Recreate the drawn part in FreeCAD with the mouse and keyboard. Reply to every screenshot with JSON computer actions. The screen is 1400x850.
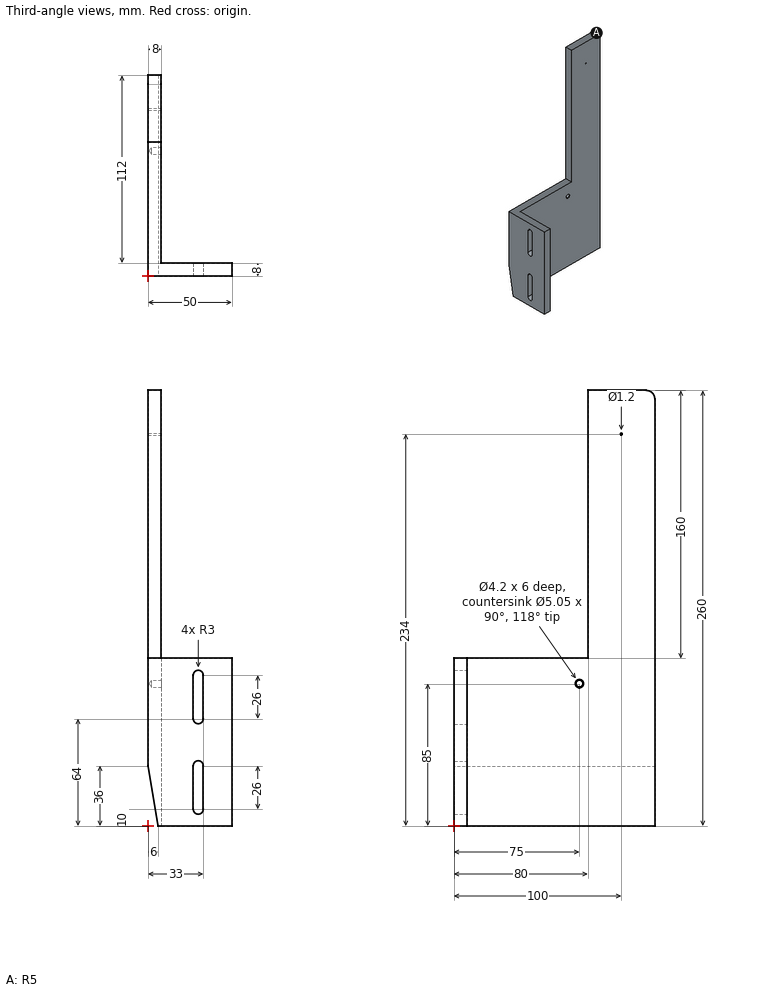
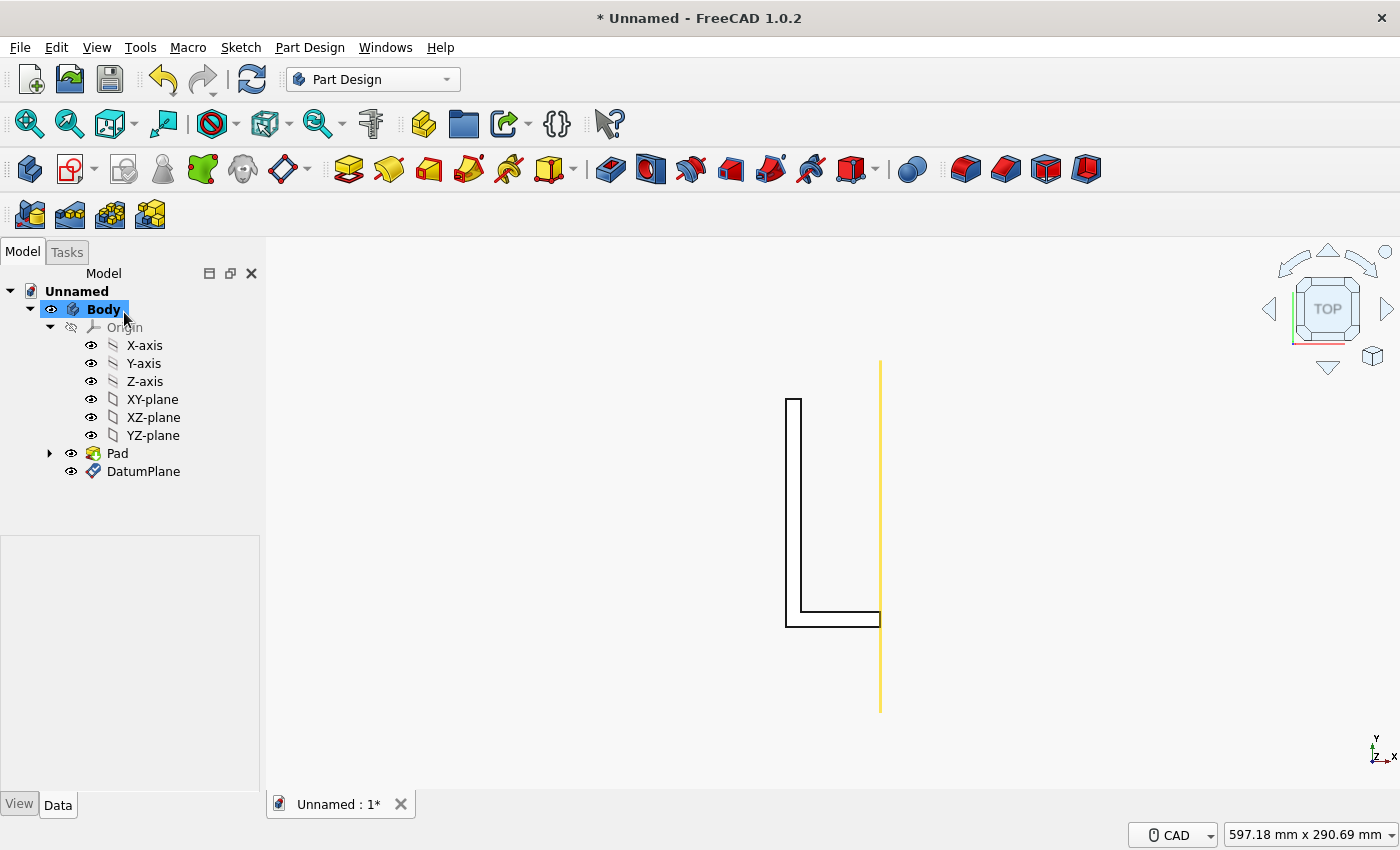
{"action": "left_click", "coordinate": [116, 471]}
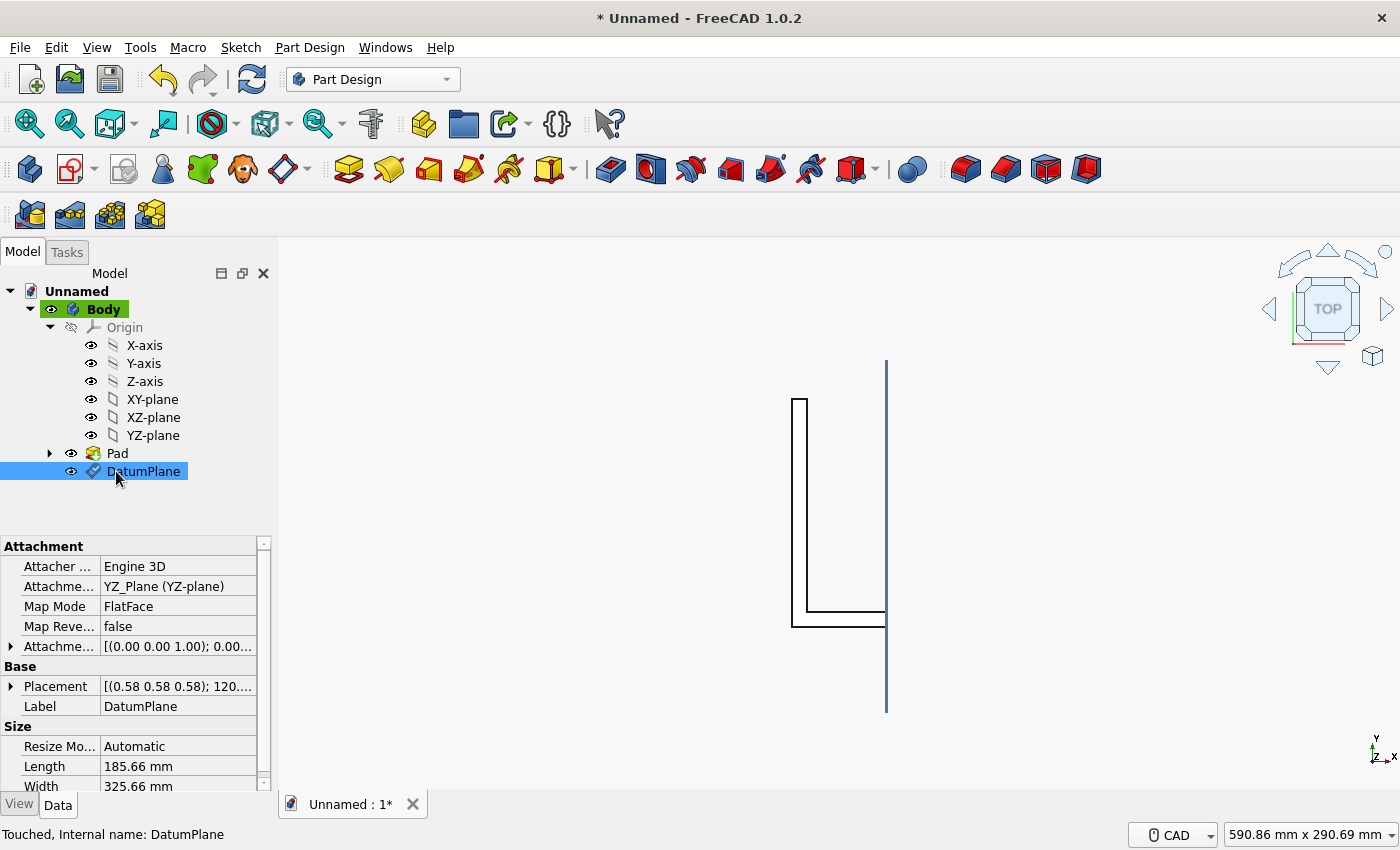
{"action": "left_click", "coordinate": [70, 170]}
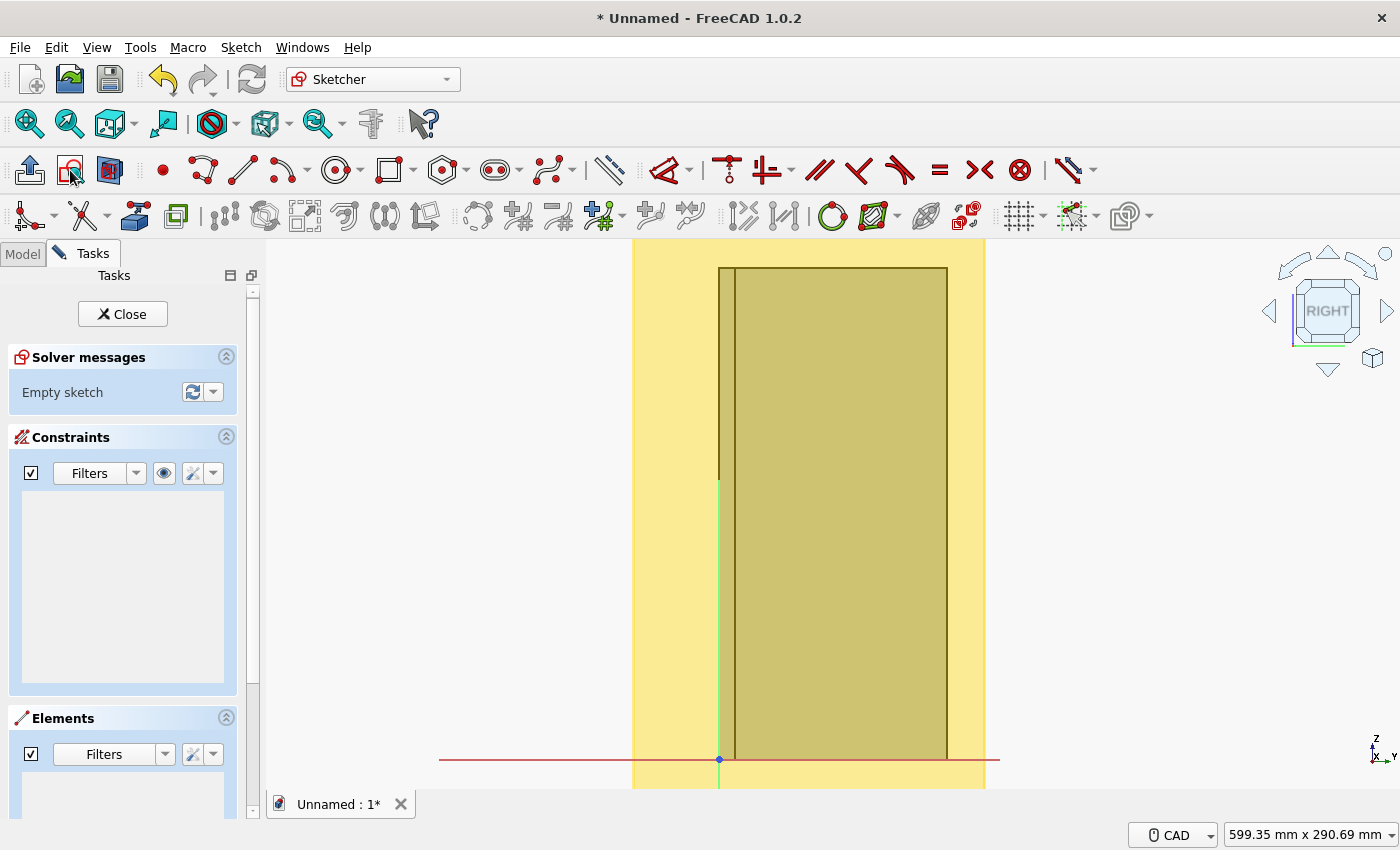
{"action": "scroll", "coordinate": [702, 514], "scroll_direction": "down", "scroll_amount": 2}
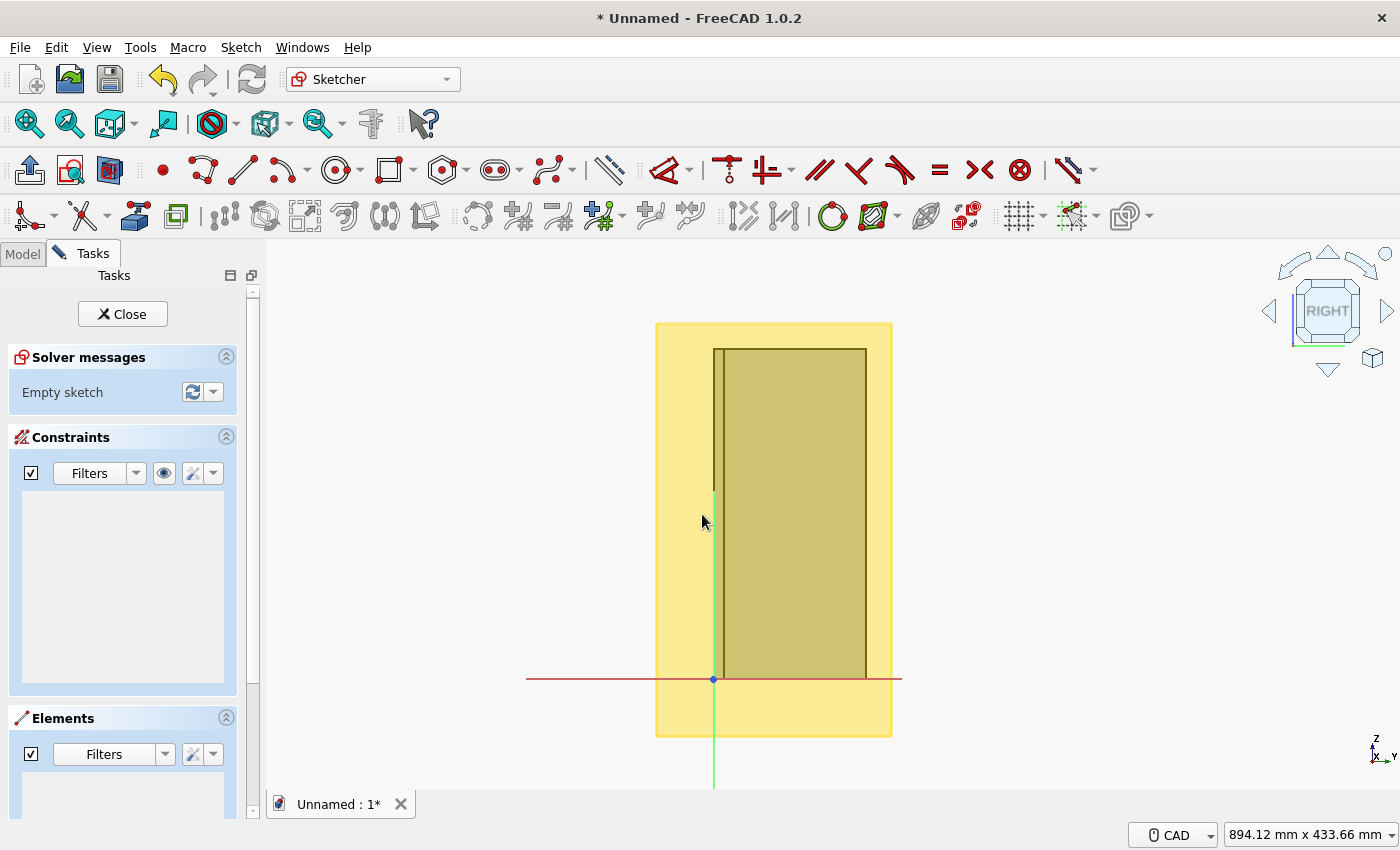
{"action": "left_click", "coordinate": [390, 170]}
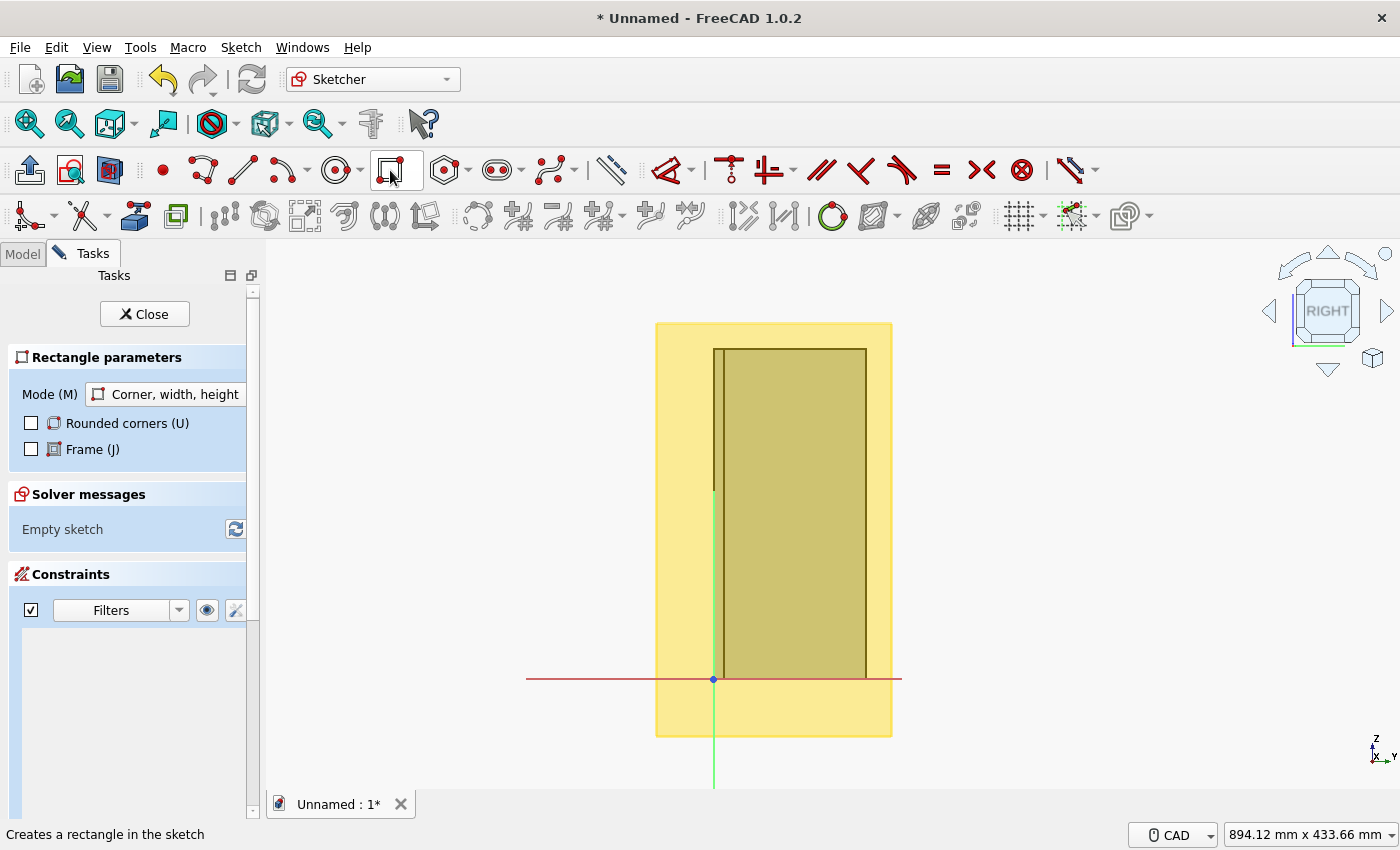
{"action": "left_click", "coordinate": [714, 349]}
{"action": "mouse_move", "coordinate": [815, 552]}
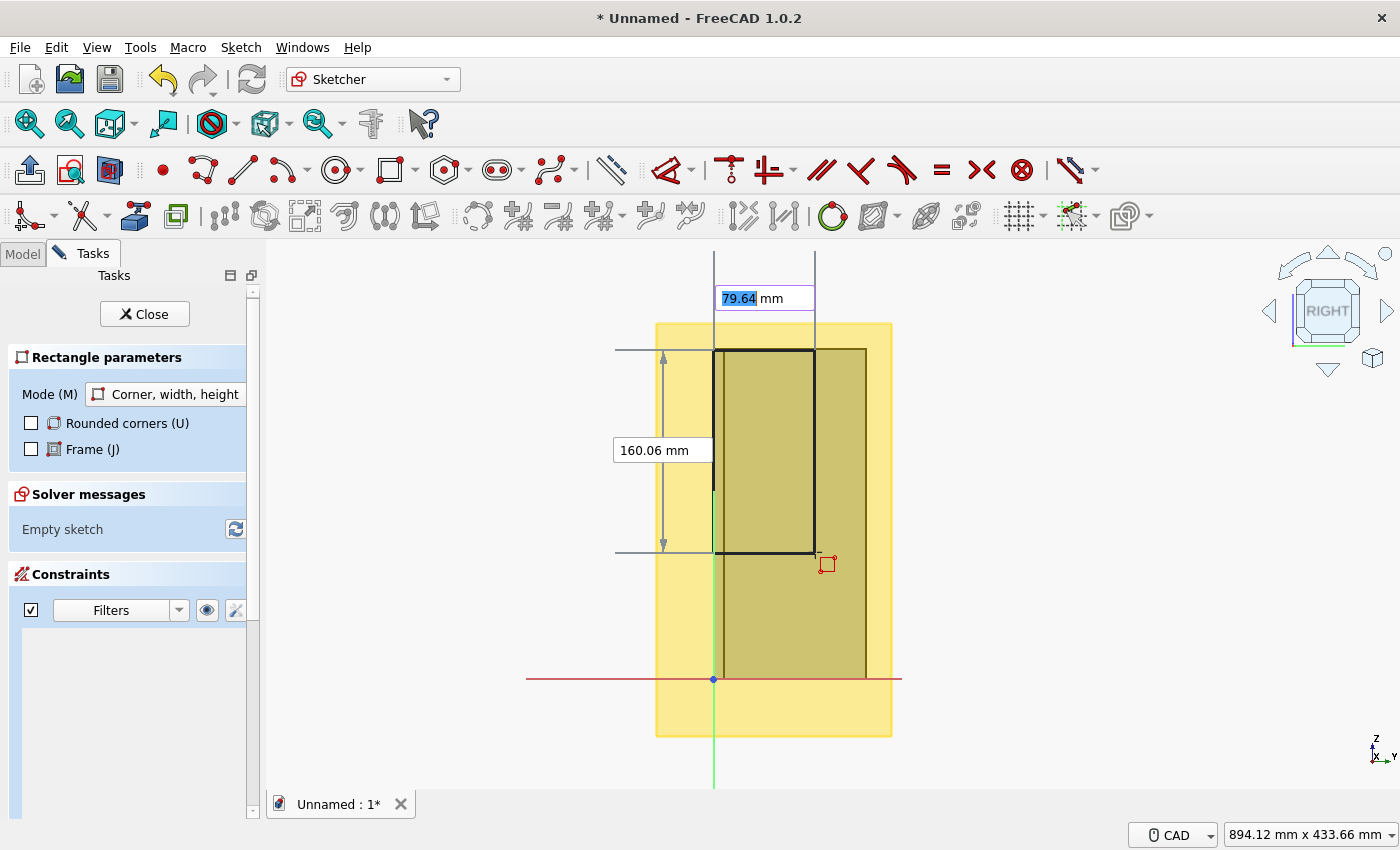
{"action": "type", "text": "80"}
{"action": "key", "text": "Tab"}
{"action": "type", "text": "160"}
{"action": "key", "text": "Return"}
{"action": "key", "text": "Escape"}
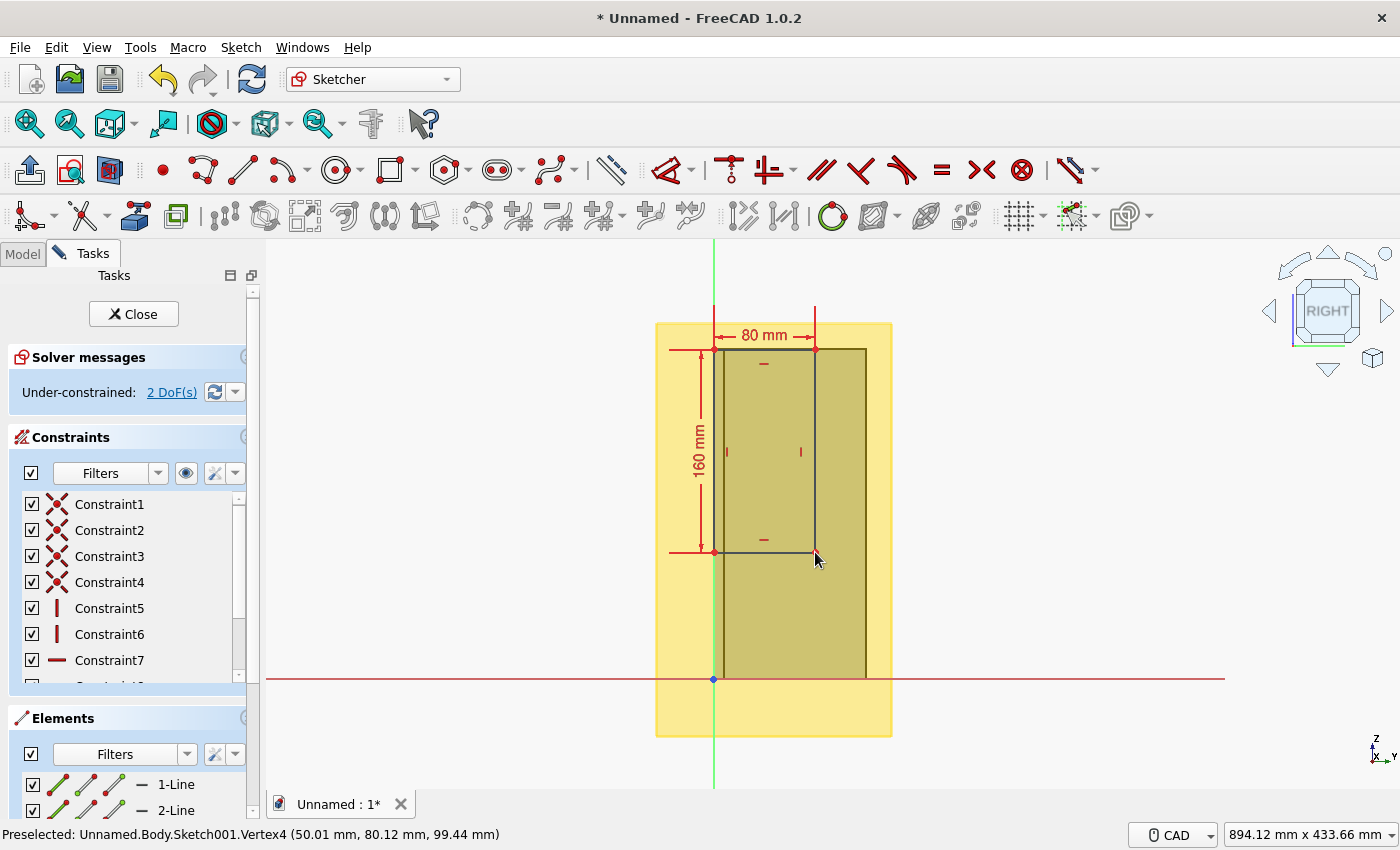
{"action": "left_click", "coordinate": [714, 350]}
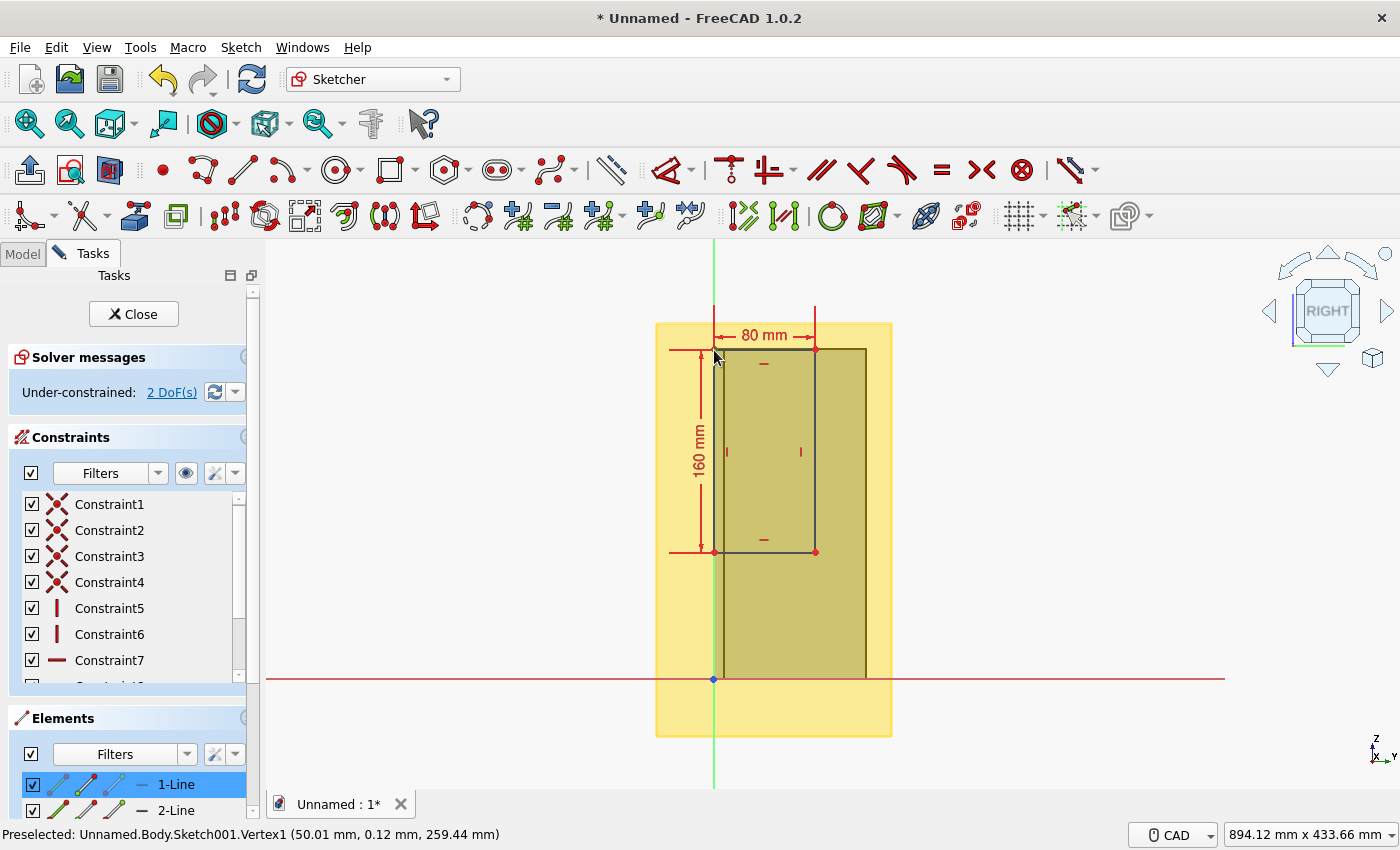
{"action": "left_click", "coordinate": [714, 726]}